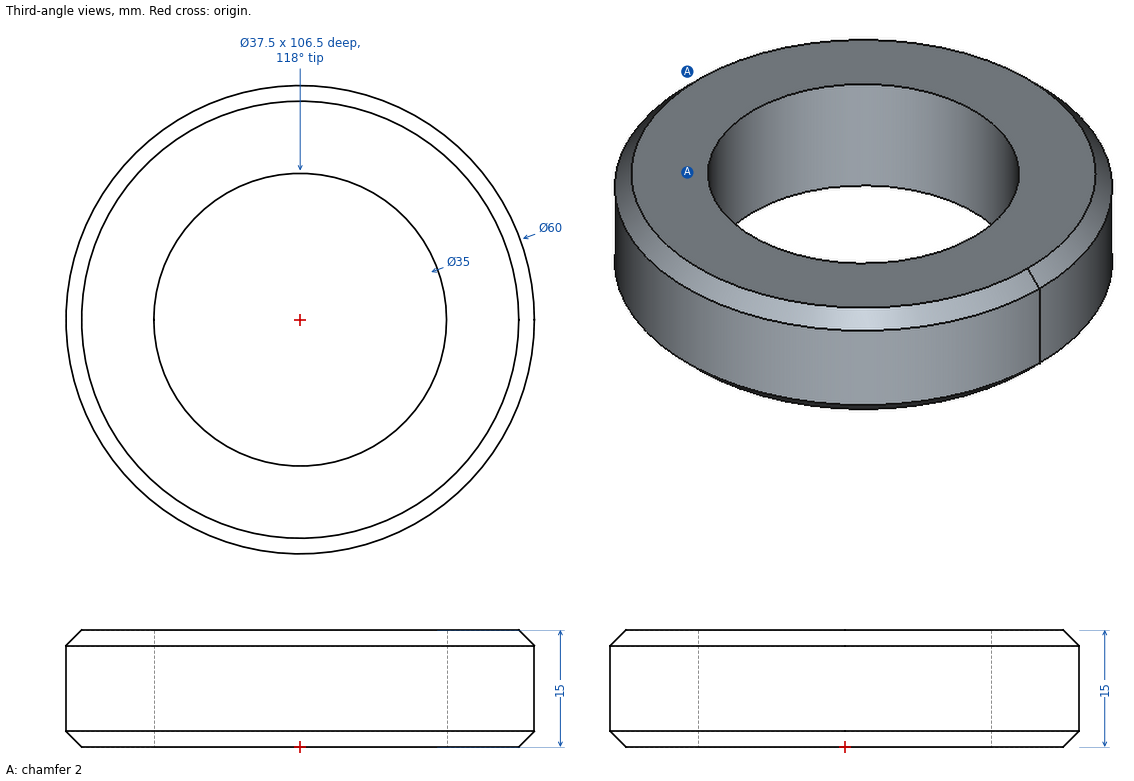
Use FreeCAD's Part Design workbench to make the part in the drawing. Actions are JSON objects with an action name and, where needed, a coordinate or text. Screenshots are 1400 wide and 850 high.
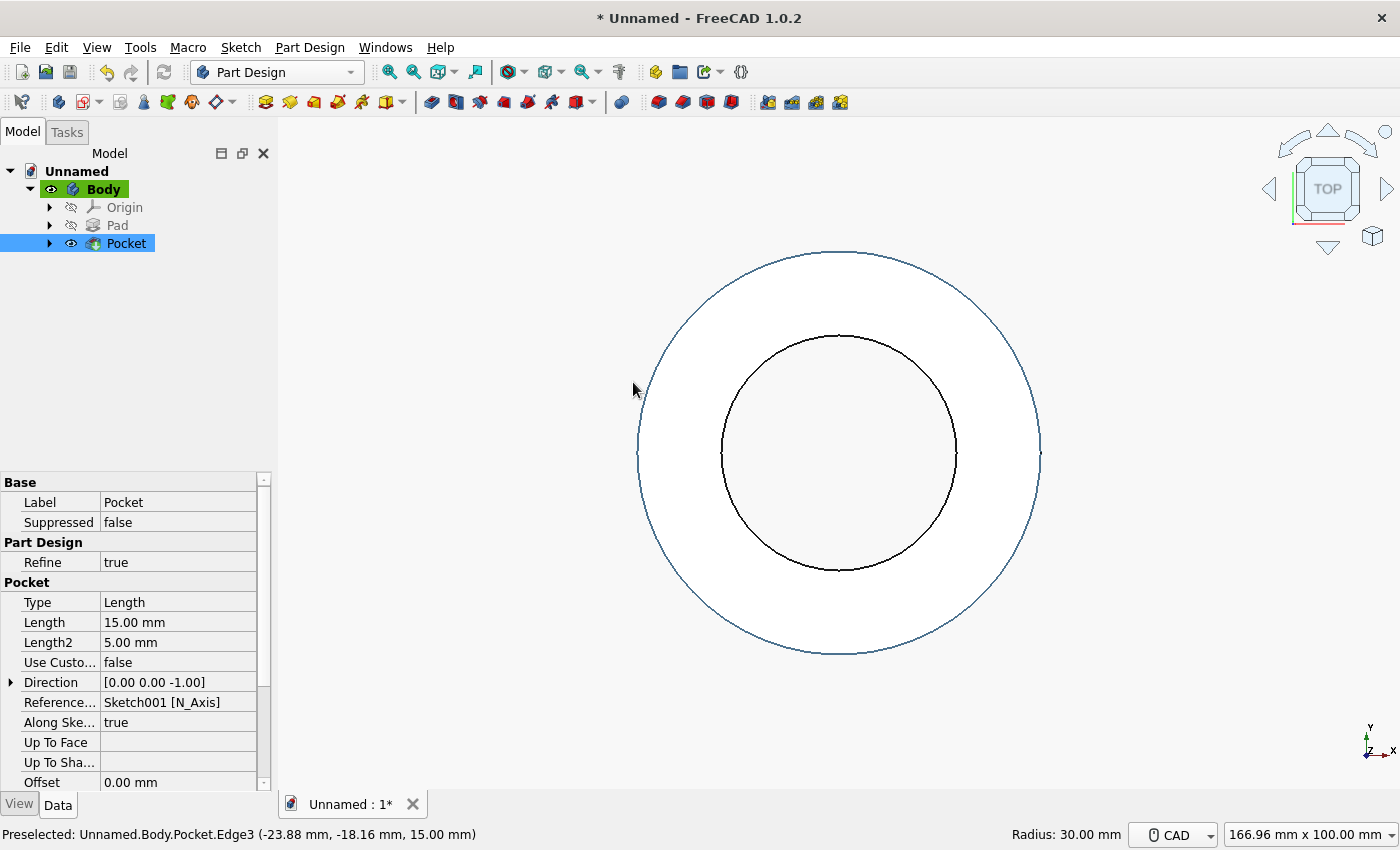
{"action": "key", "text": "1"}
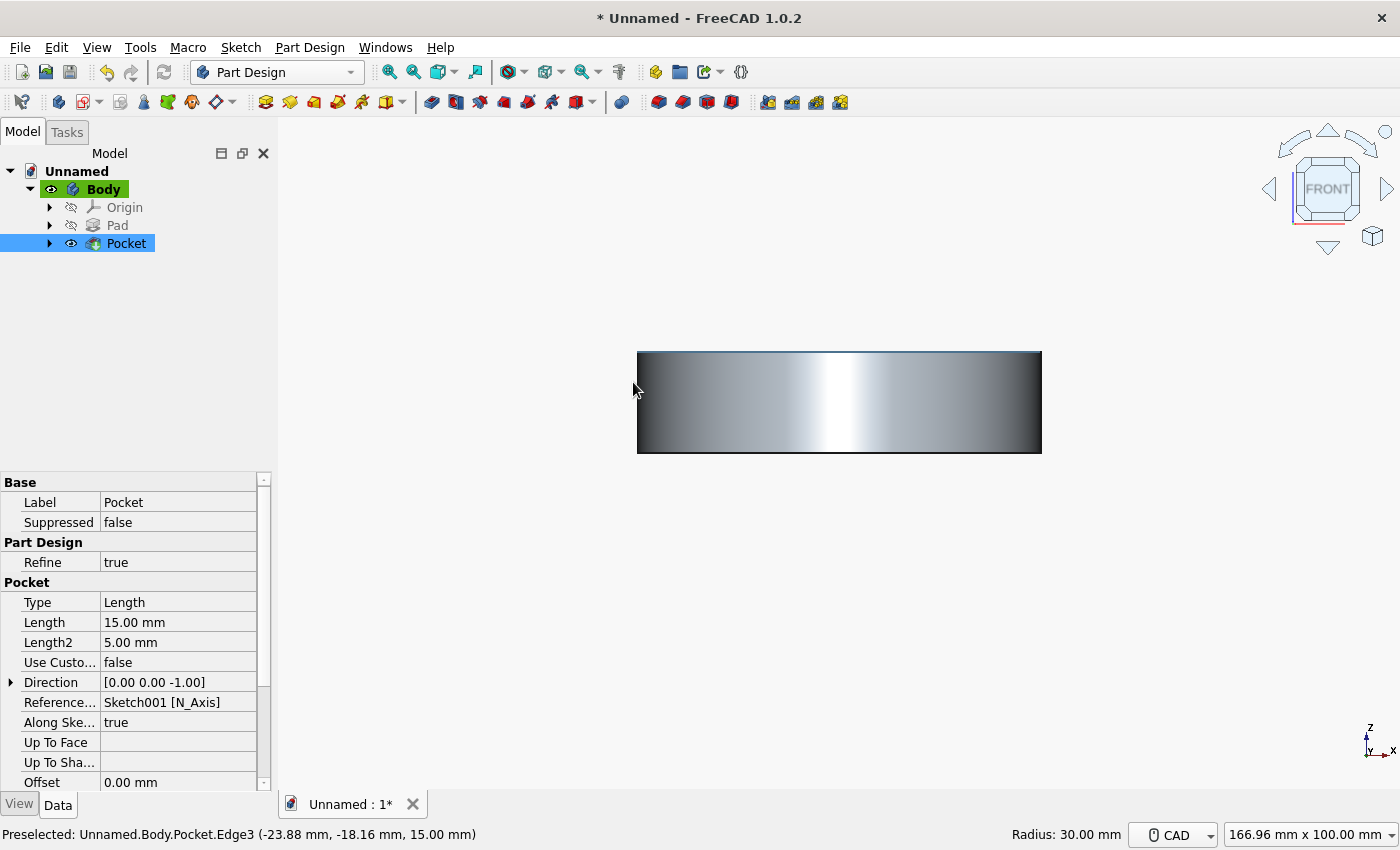
{"action": "left_click", "coordinate": [390, 72]}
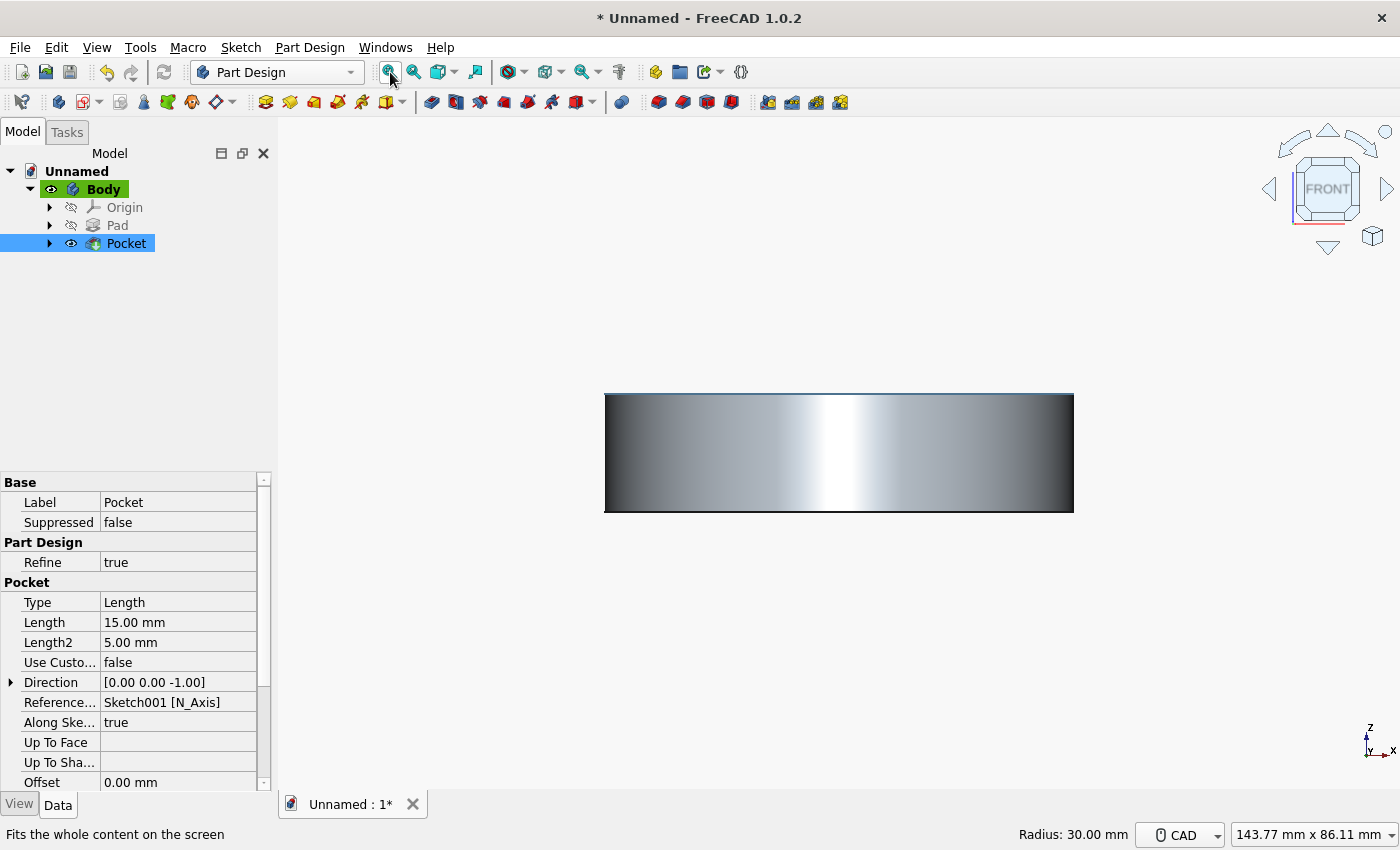
{"action": "left_click", "coordinate": [650, 511], "text": "ctrl"}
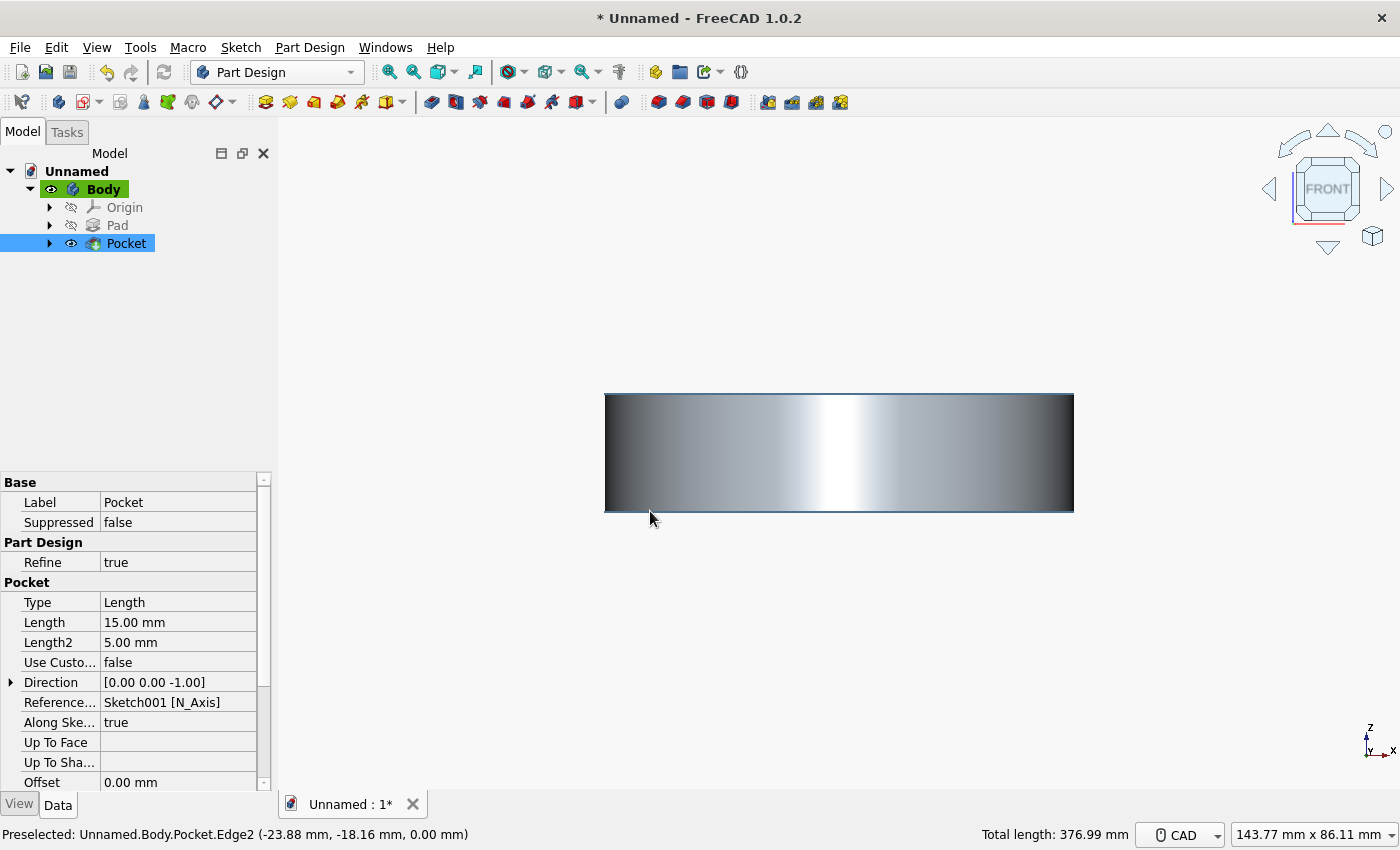
{"action": "left_click", "coordinate": [684, 102]}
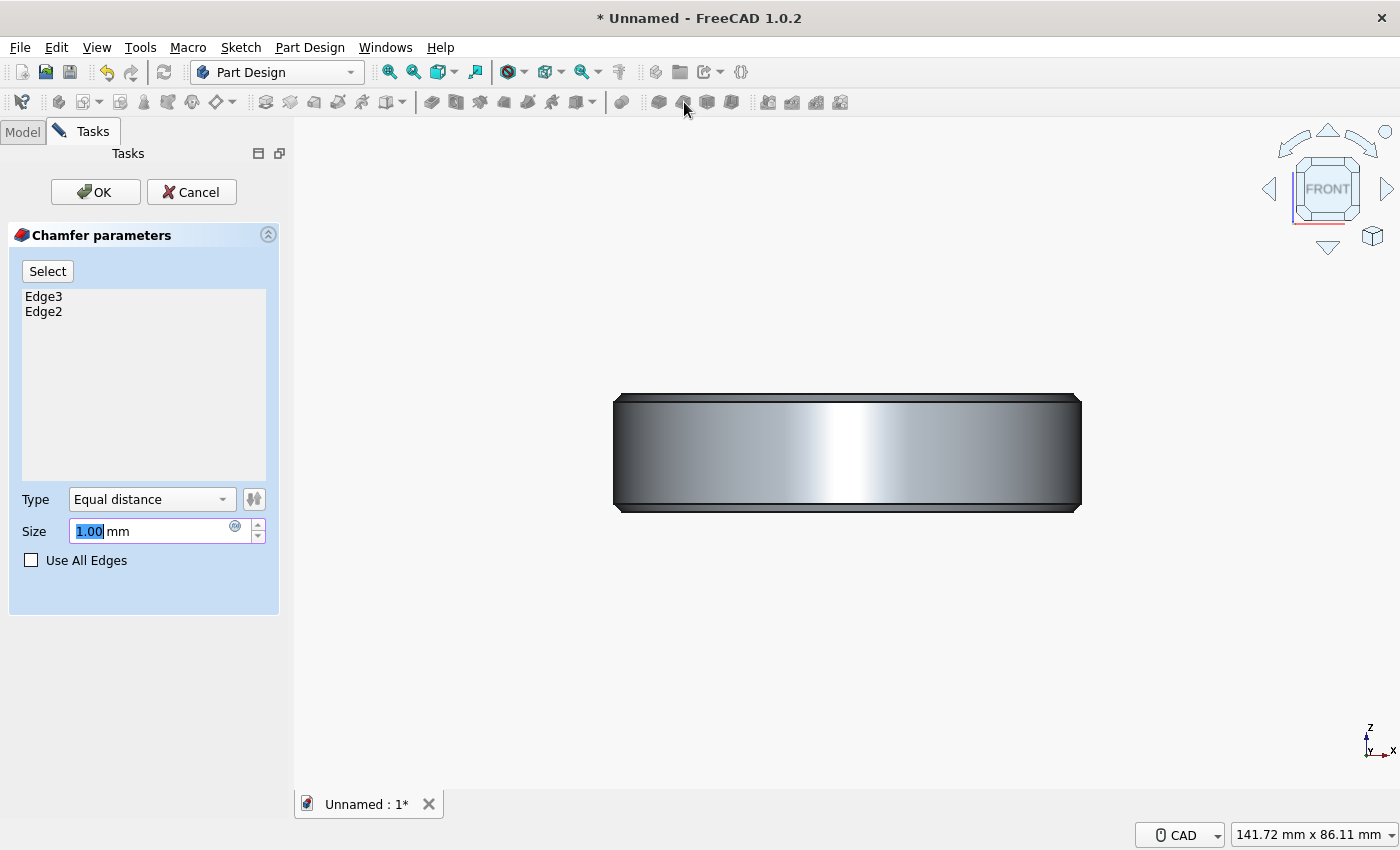
{"action": "type", "text": "2"}
{"action": "key", "text": "Tab"}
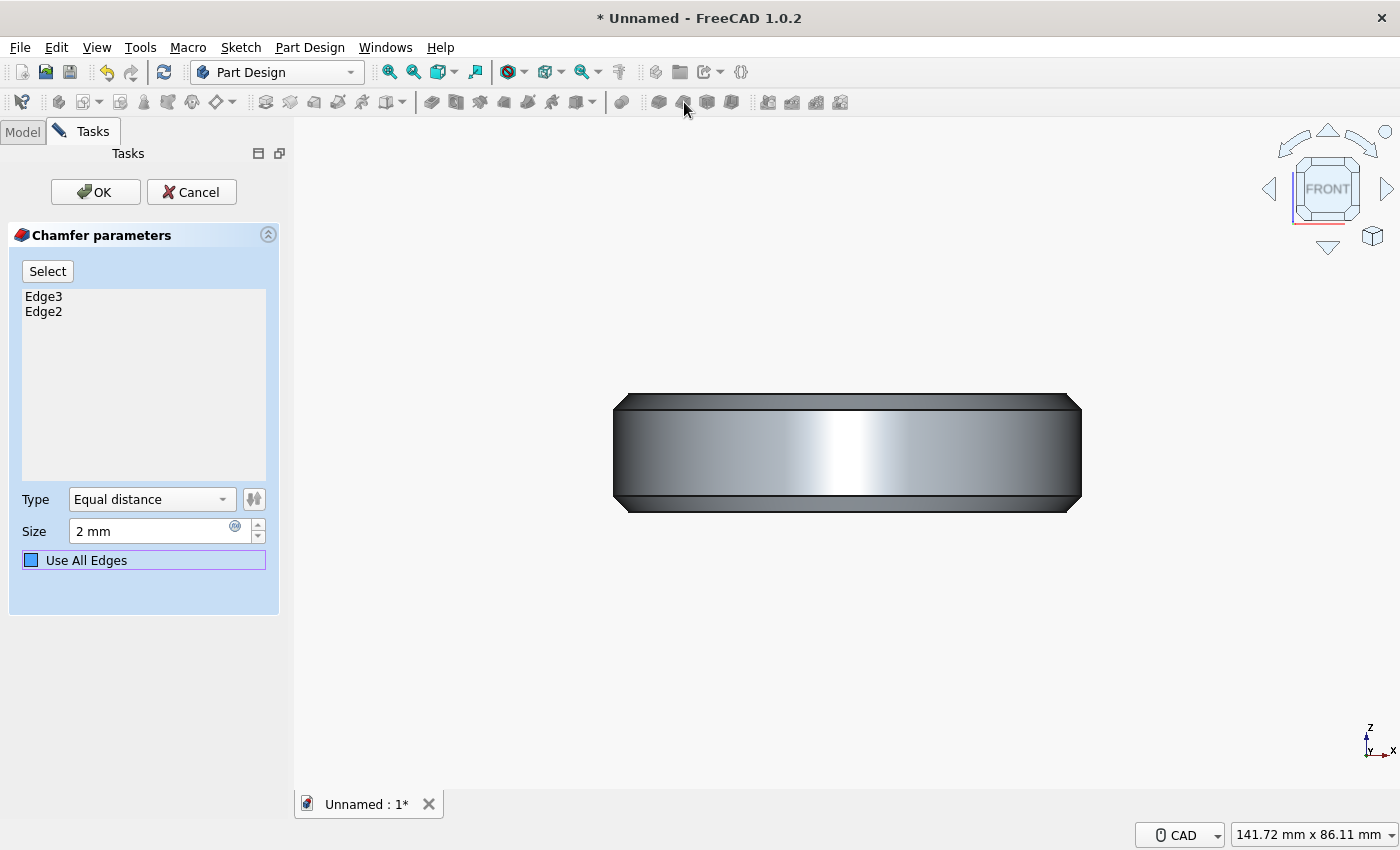
{"action": "left_click", "coordinate": [96, 192]}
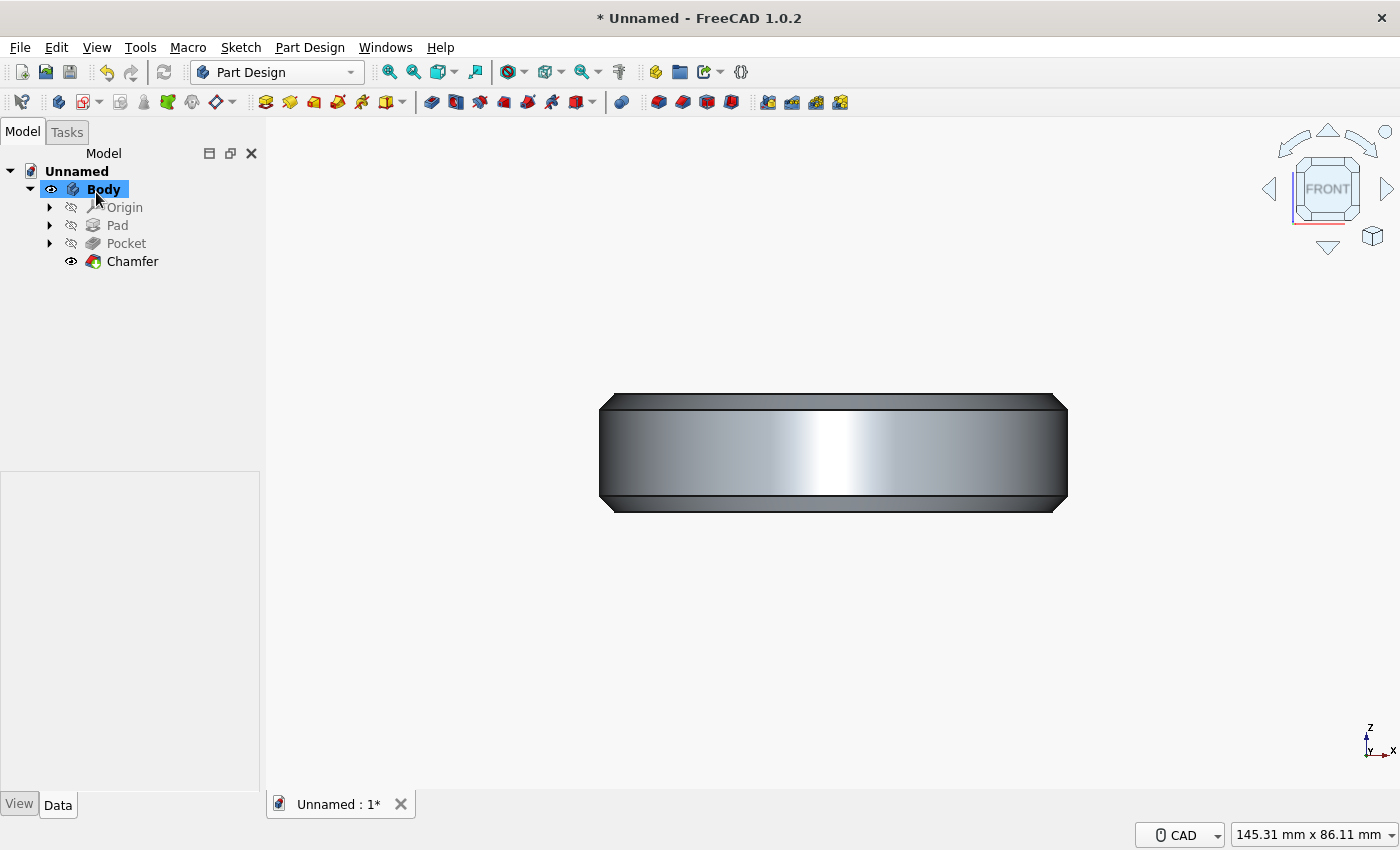
{"action": "left_click", "coordinate": [390, 72]}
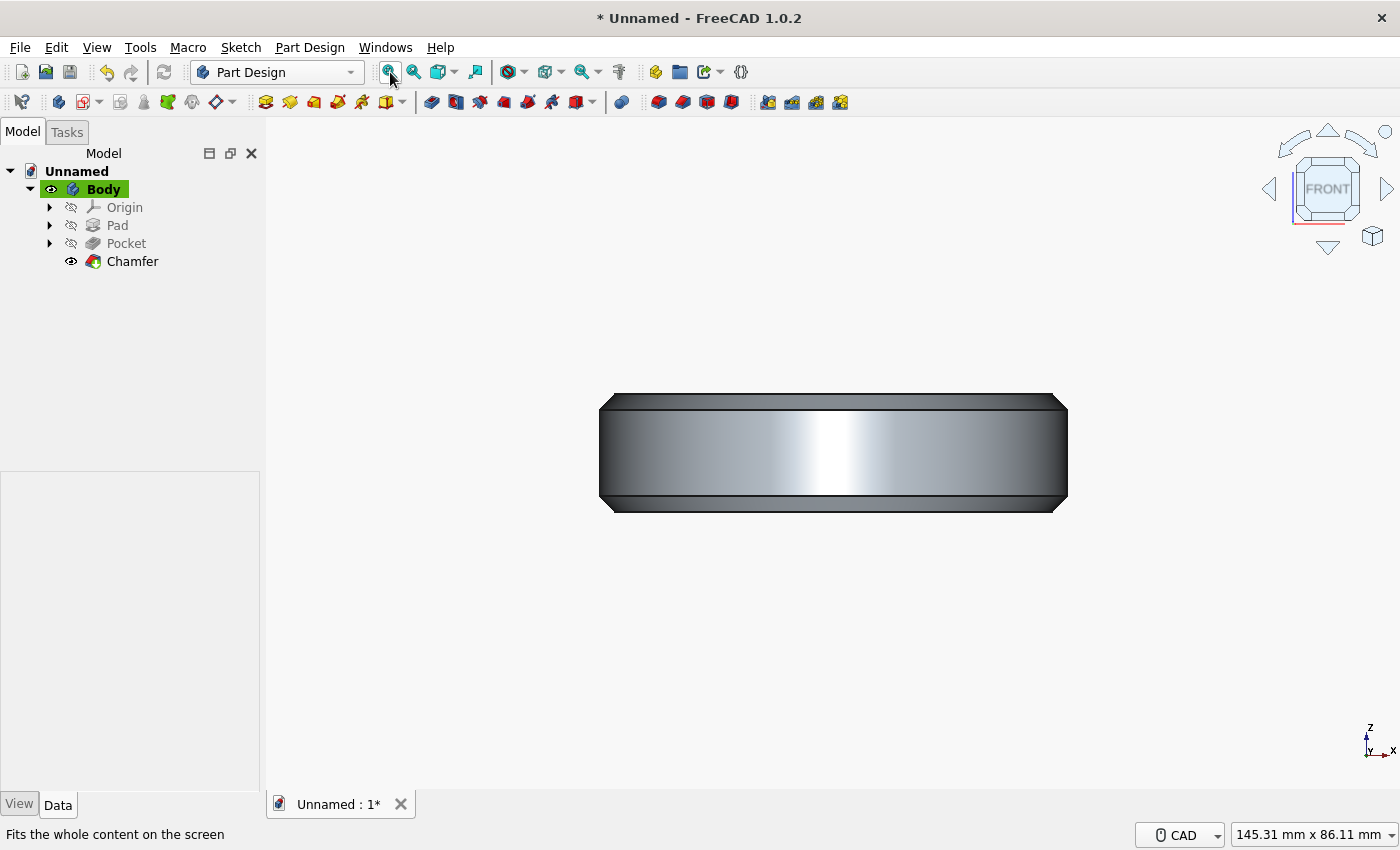
{"action": "key", "text": "0"}